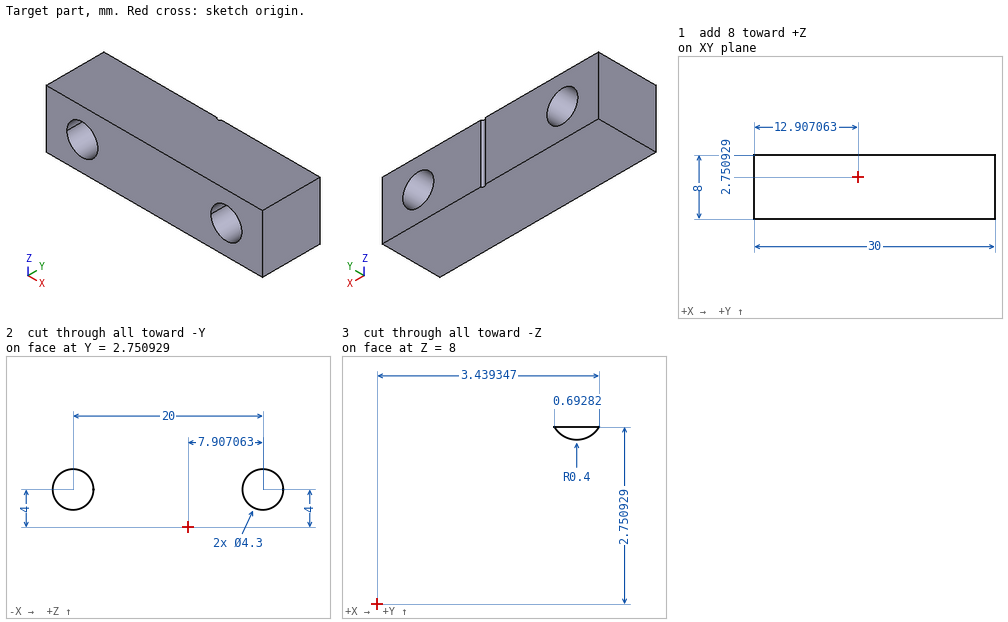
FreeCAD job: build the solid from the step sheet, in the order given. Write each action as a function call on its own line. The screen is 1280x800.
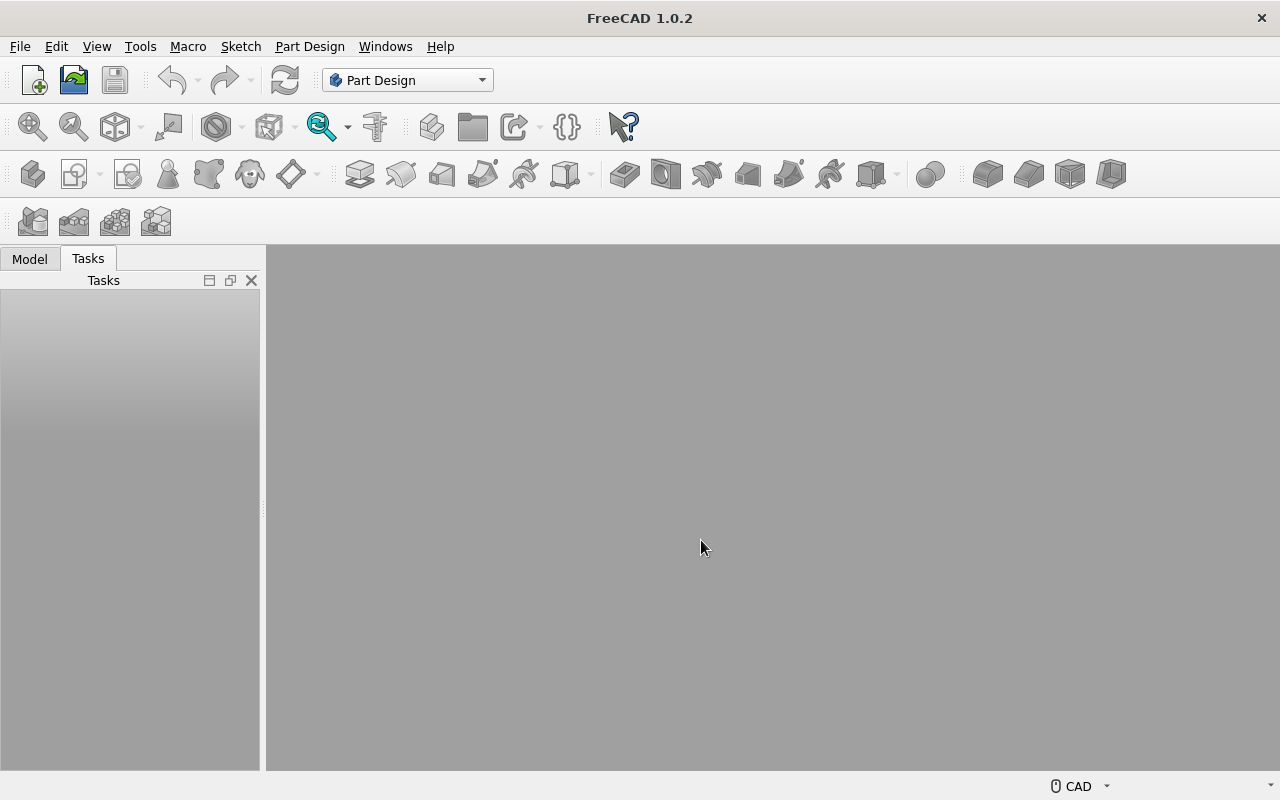
key(ctrl+n)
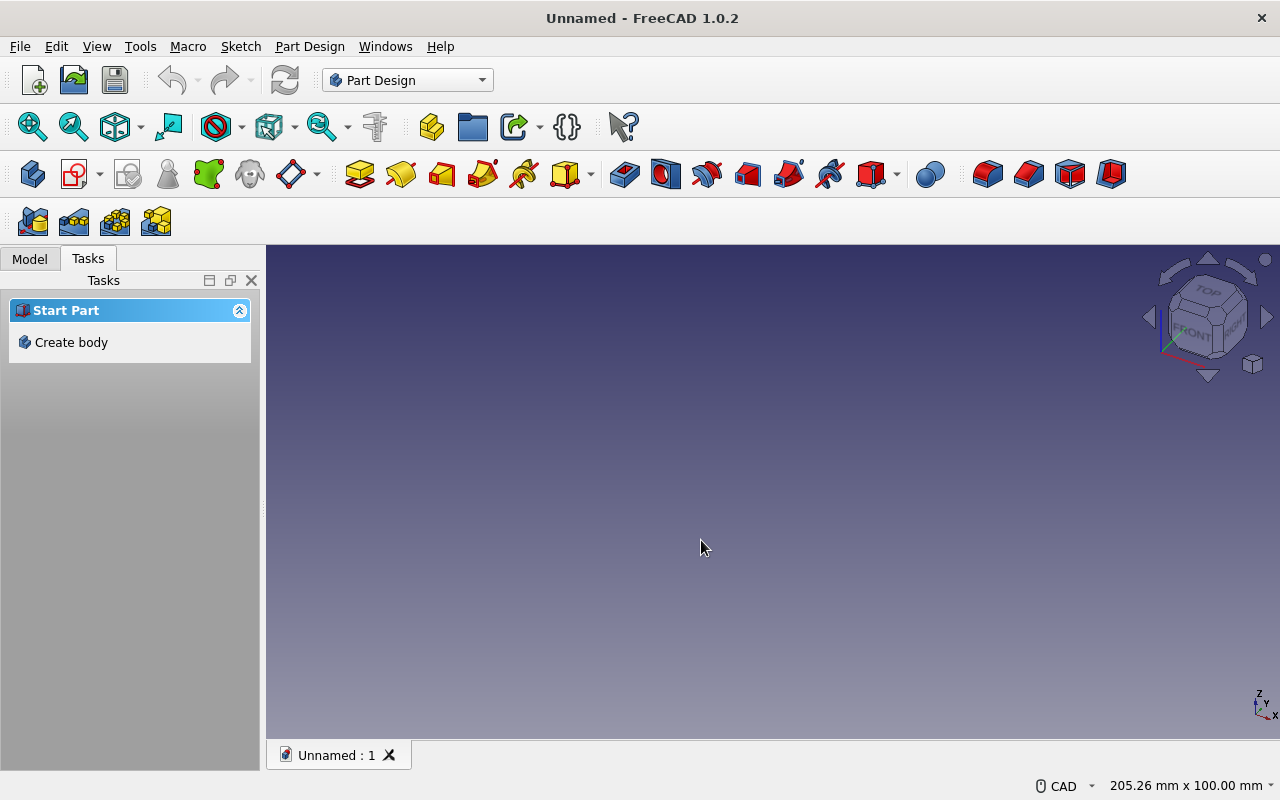
click(74, 174)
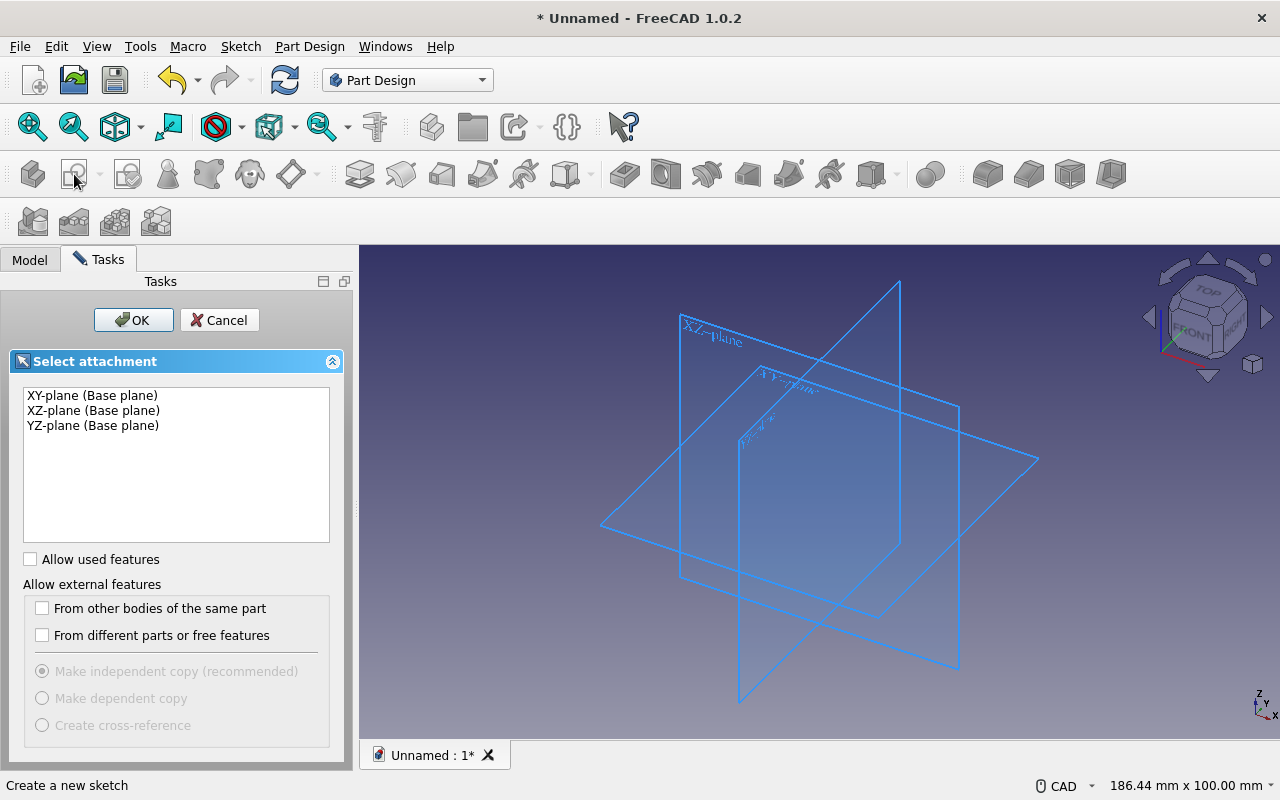
click(84, 396)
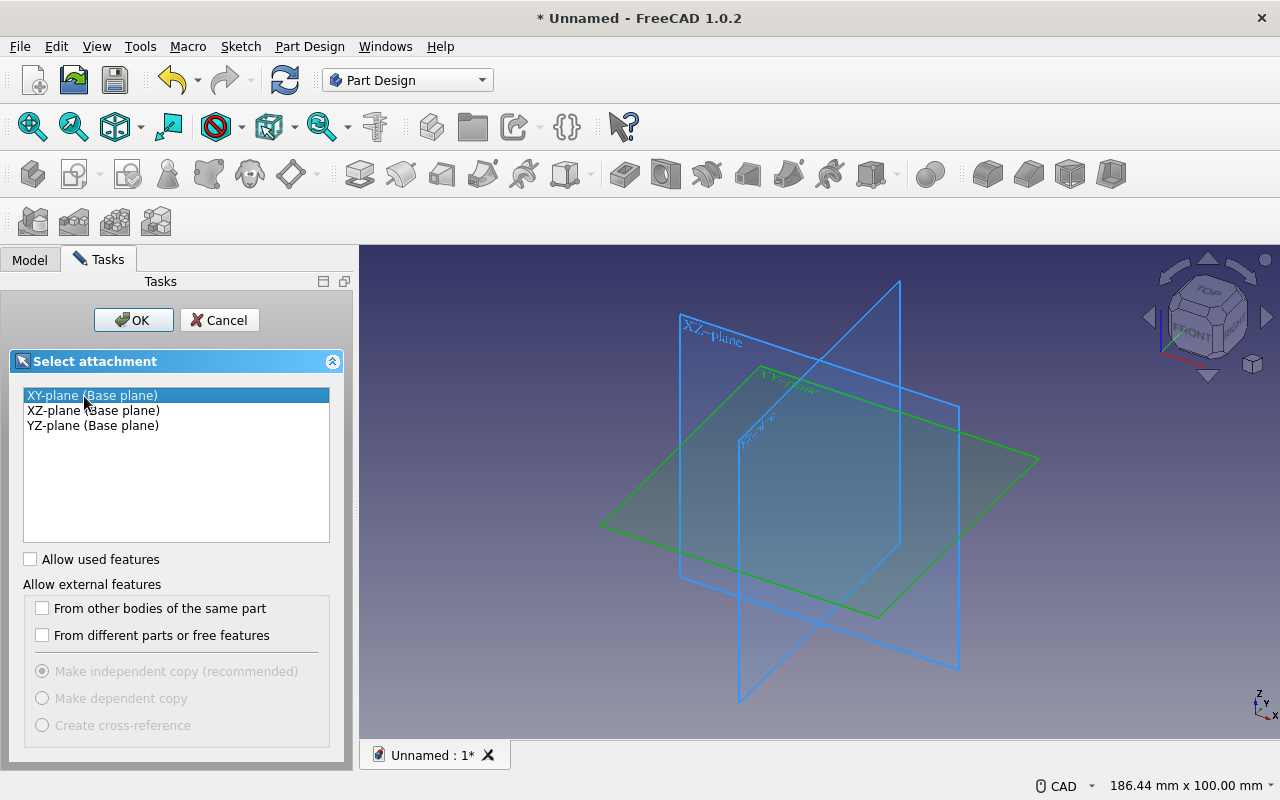
click(134, 320)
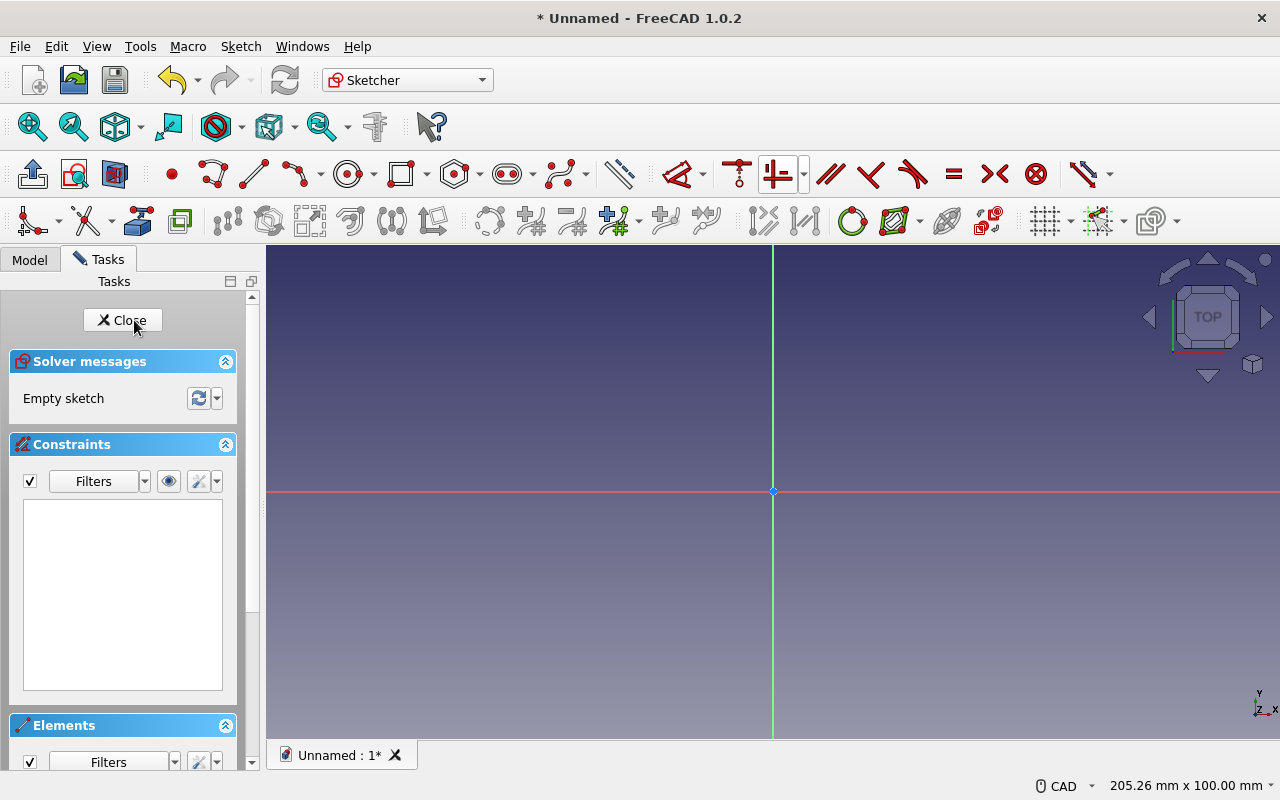
scroll(809, 500, up, 7)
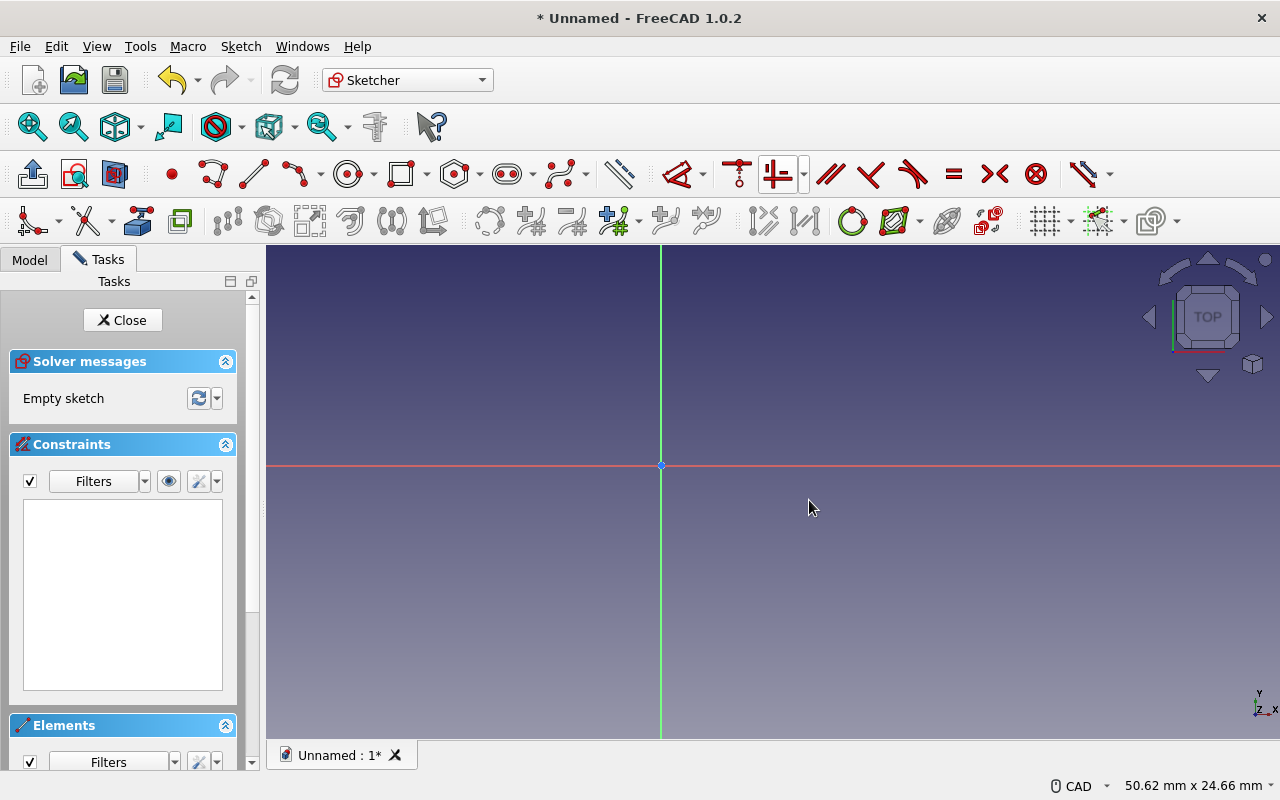
key(g)
key(r)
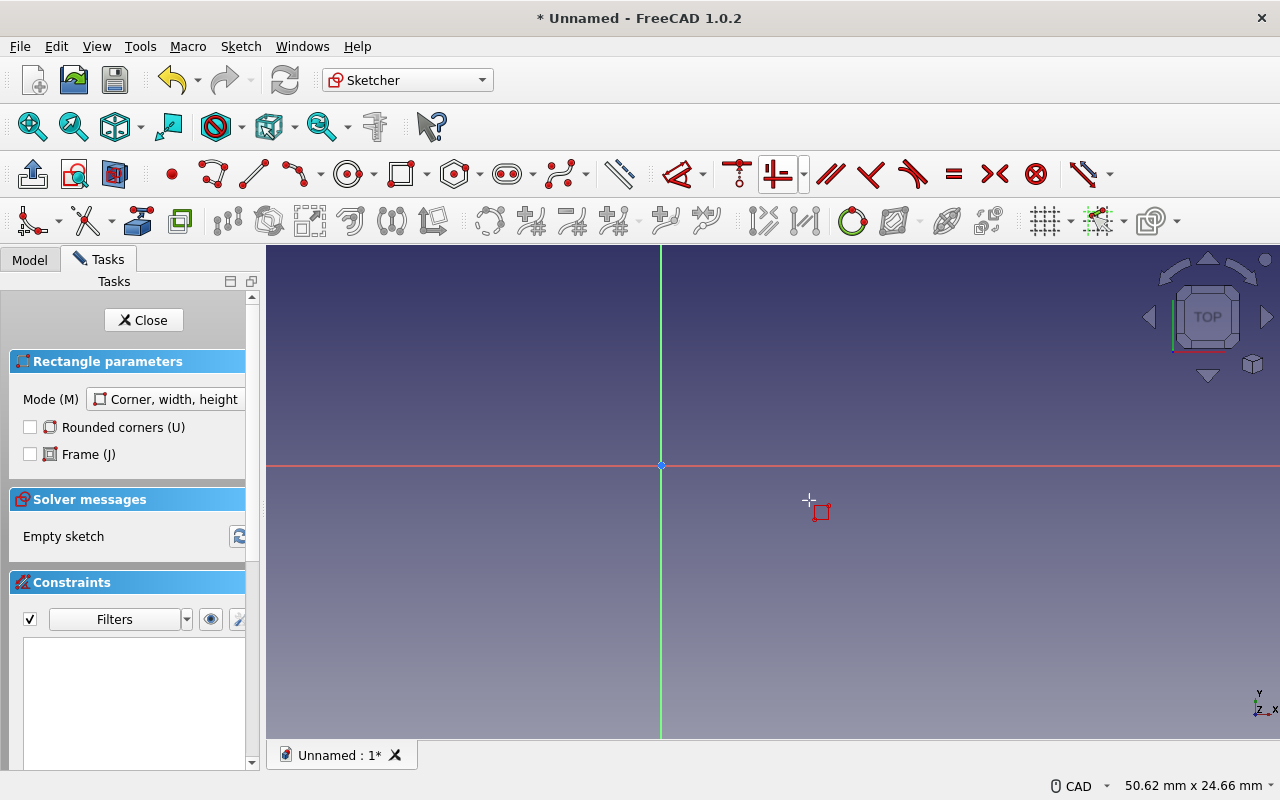
click(403, 411)
click(1004, 571)
key(Escape)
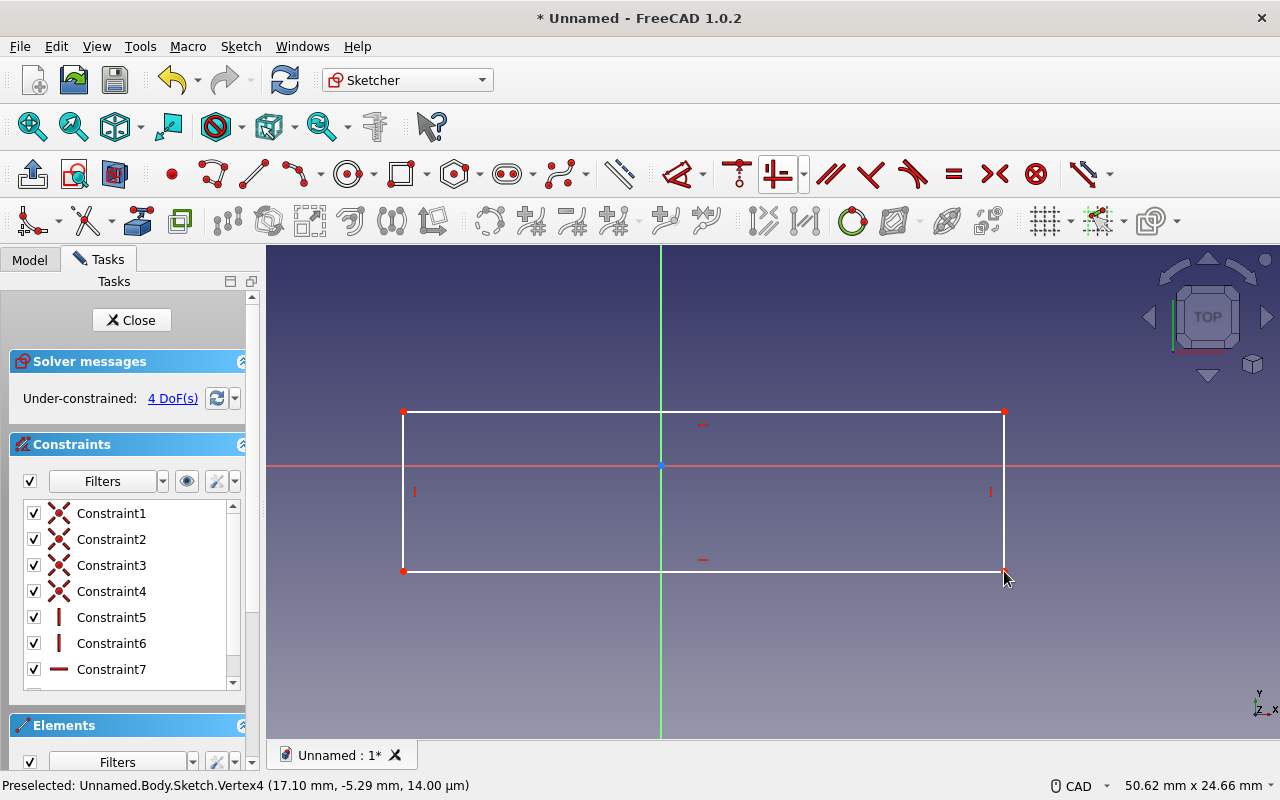
key(d)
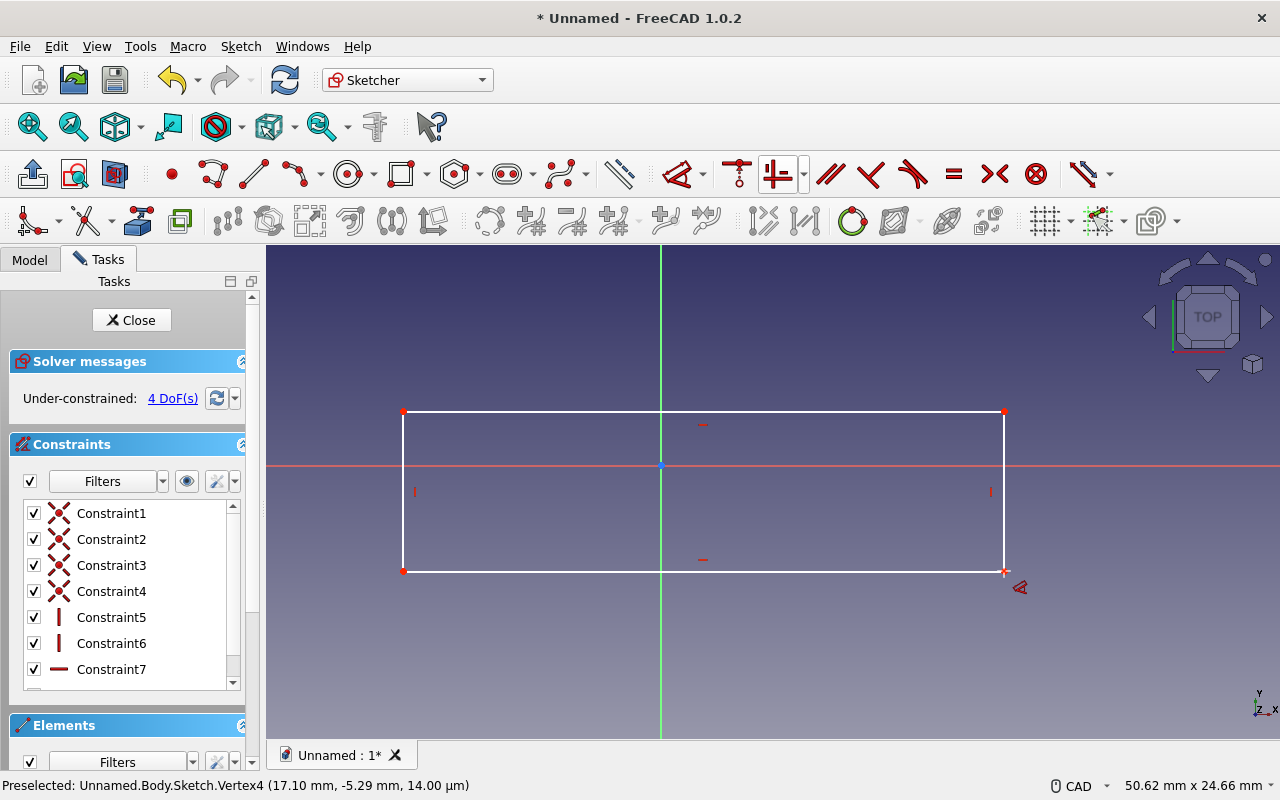
click(403, 524)
click(369, 492)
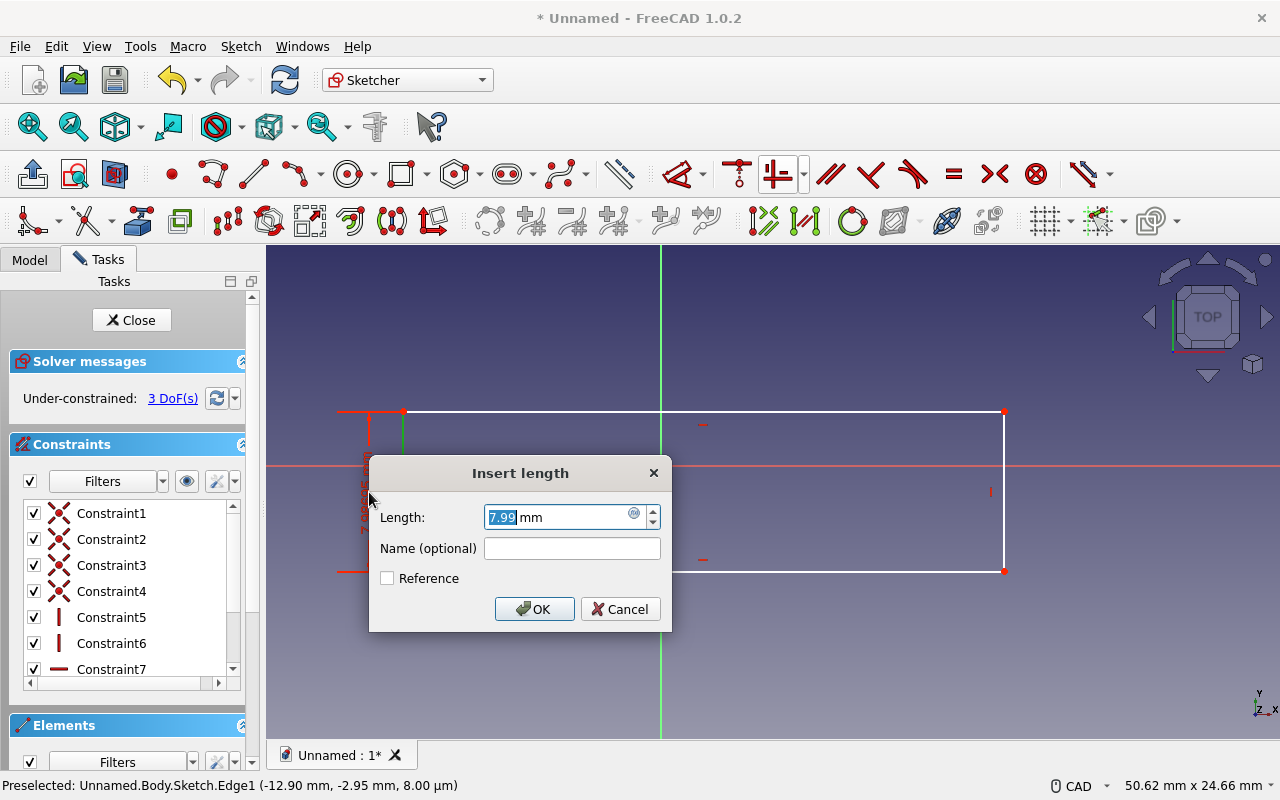
text(8)
key(Return)